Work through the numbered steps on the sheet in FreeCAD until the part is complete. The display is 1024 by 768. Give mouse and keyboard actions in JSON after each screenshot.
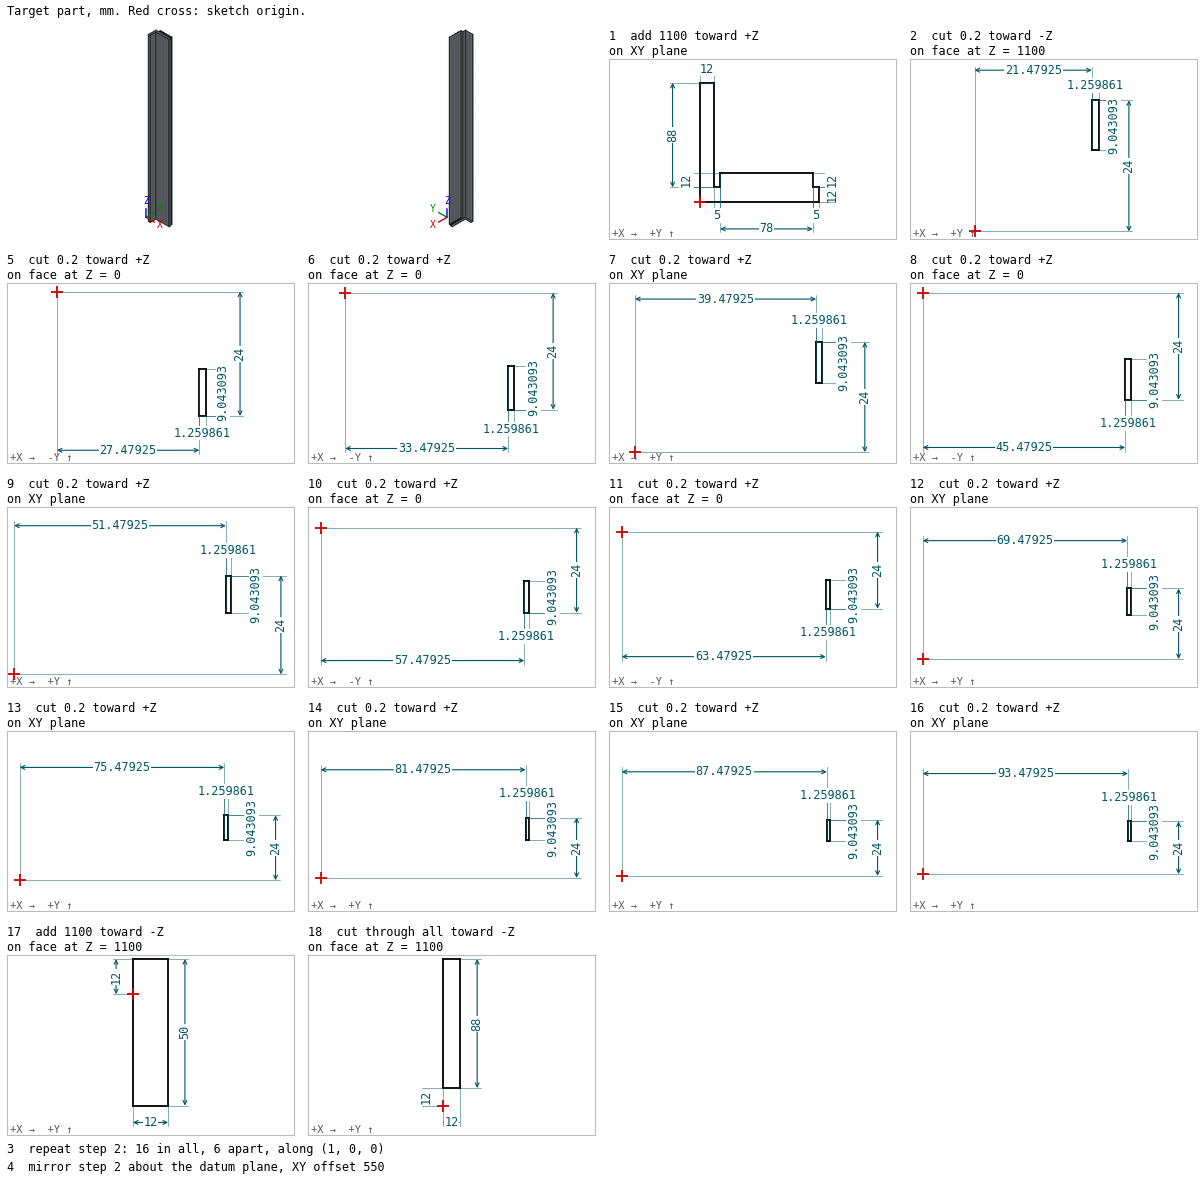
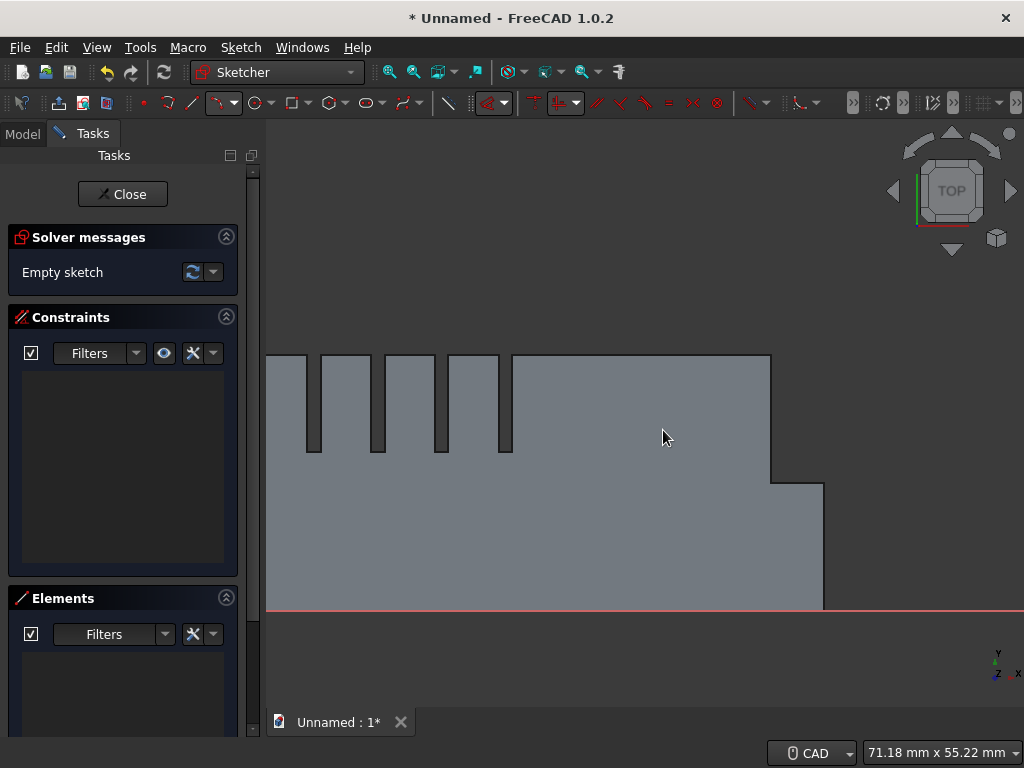
{"action": "scroll", "coordinate": [567, 400], "scroll_direction": "up", "scroll_amount": 7}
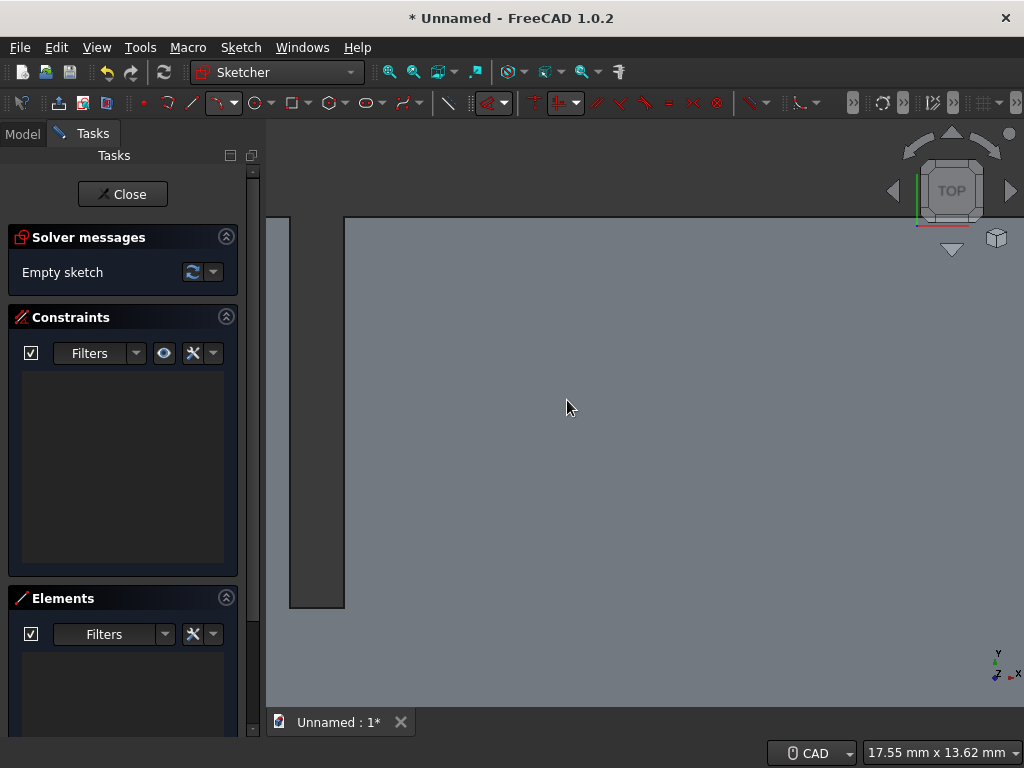
{"action": "left_click", "coordinate": [292, 104]}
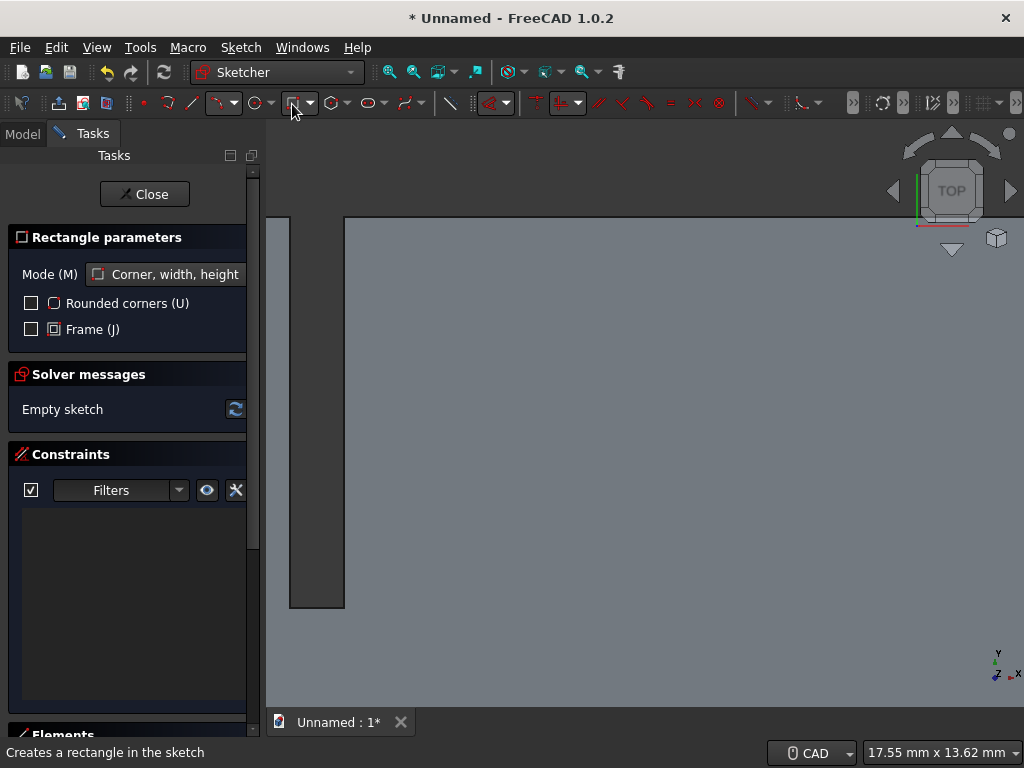
{"action": "left_click", "coordinate": [549, 217]}
{"action": "mouse_move", "coordinate": [603, 608]}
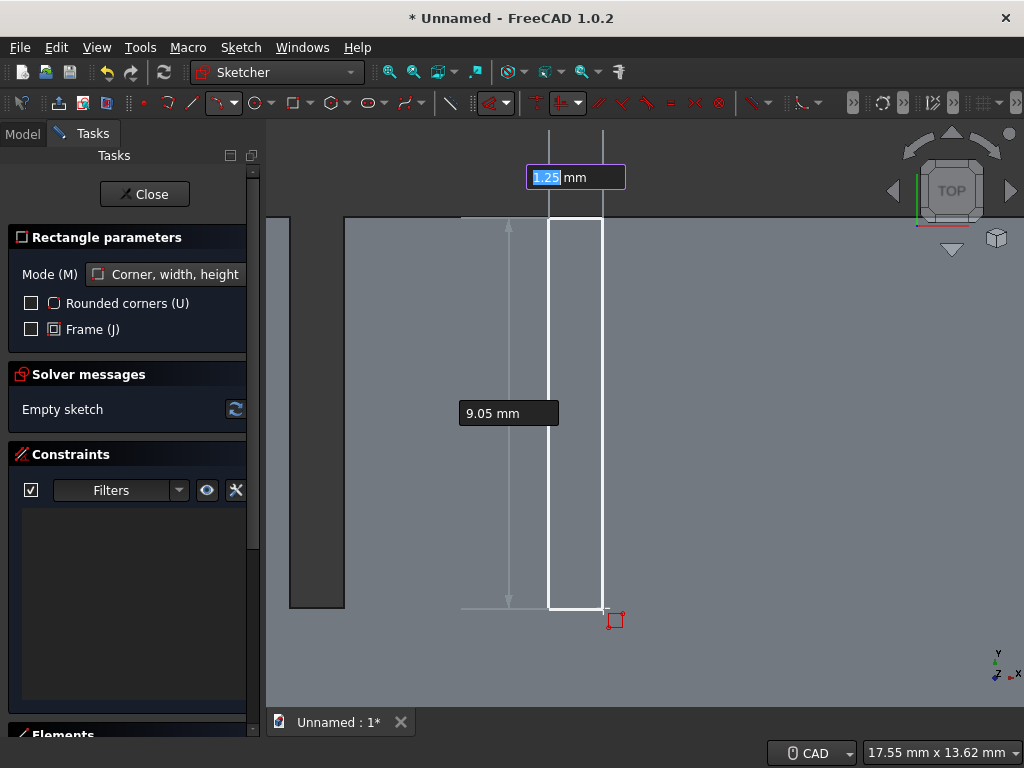
{"action": "type", "text": "1.259861"}
{"action": "key", "text": "Tab"}
{"action": "type", "text": "9.043093"}
{"action": "key", "text": "Return"}
{"action": "key", "text": "Escape"}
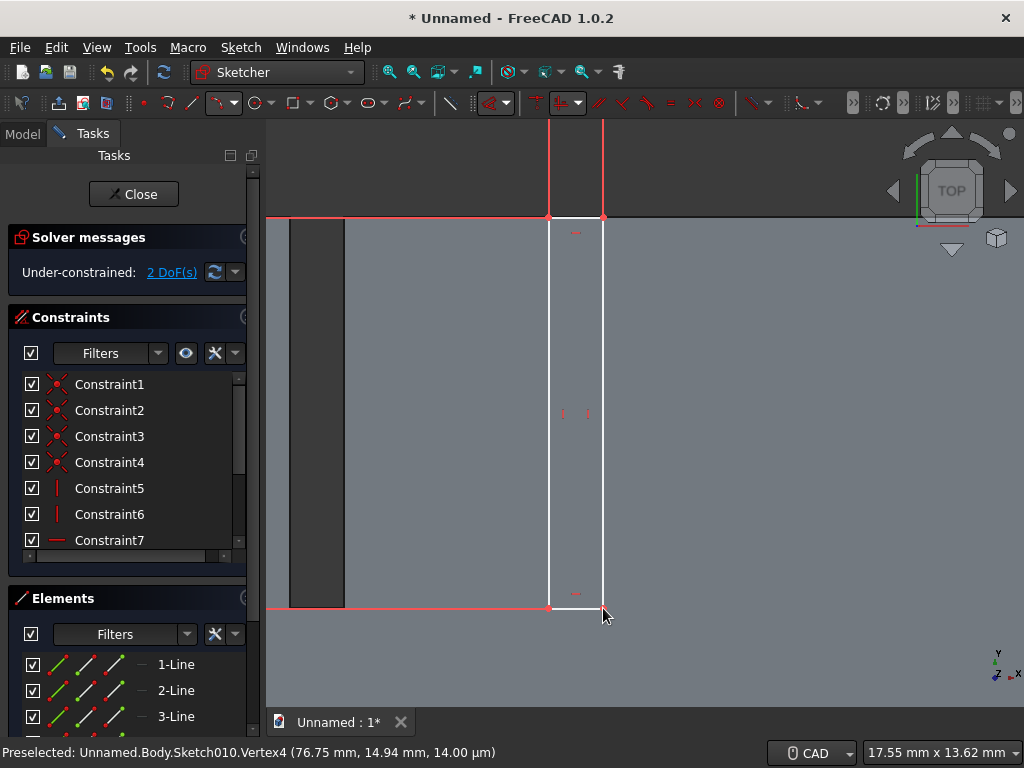
{"action": "left_click", "coordinate": [549, 218]}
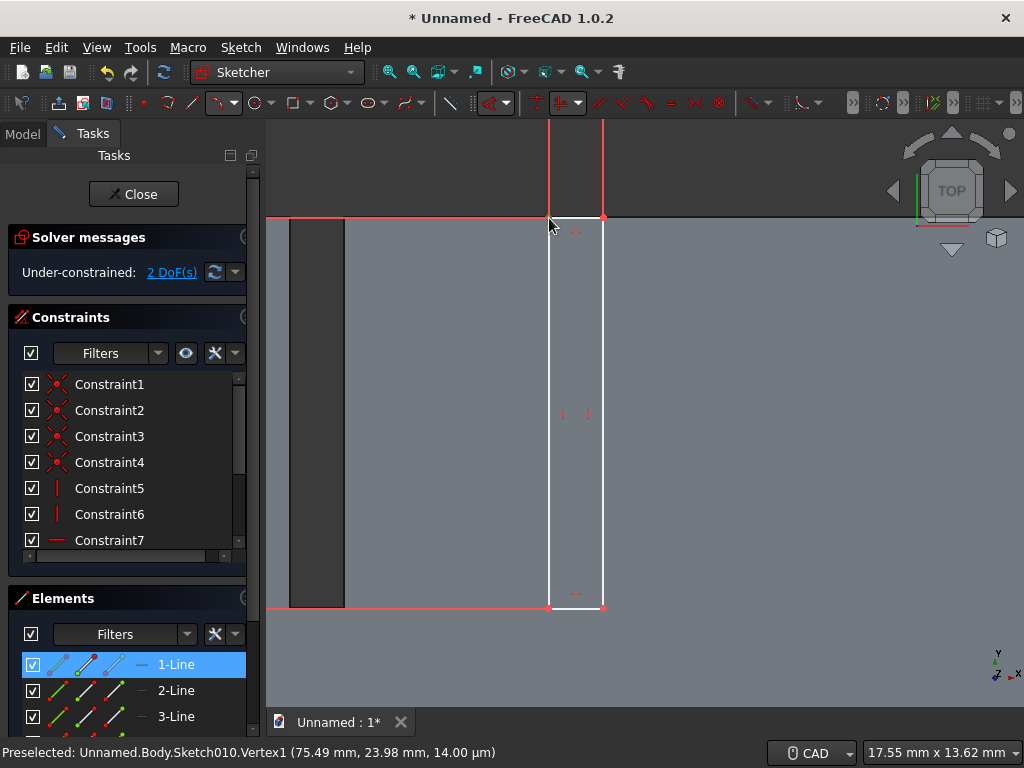
{"action": "key", "text": "i"}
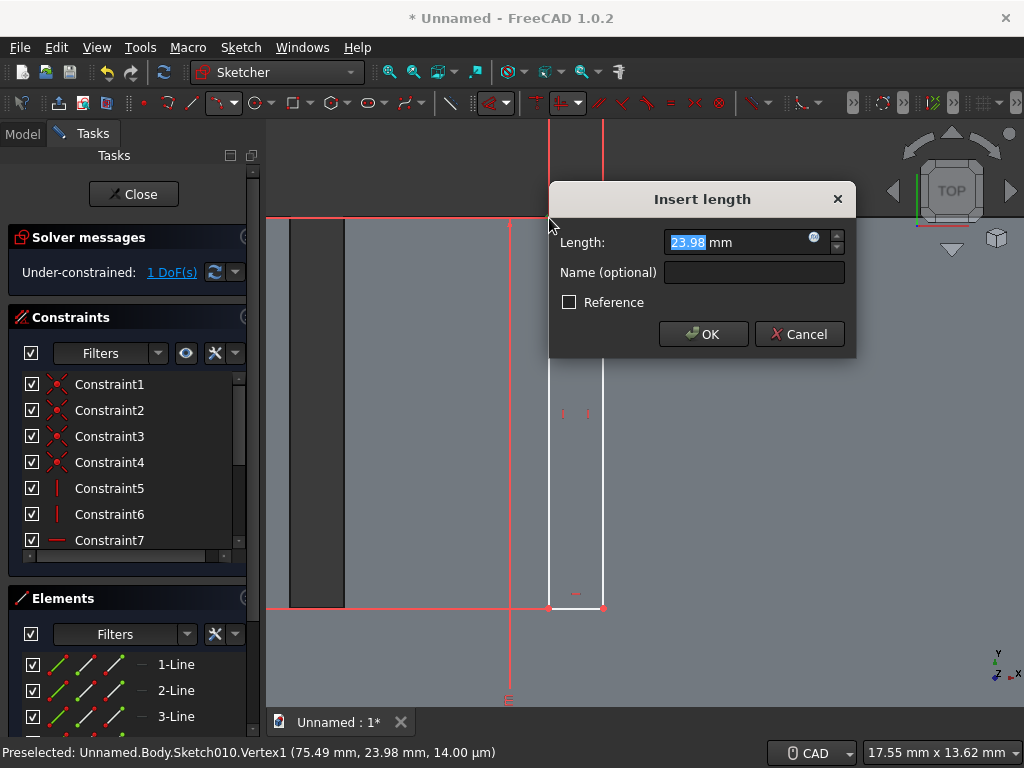
{"action": "type", "text": "24"}
{"action": "key", "text": "Return"}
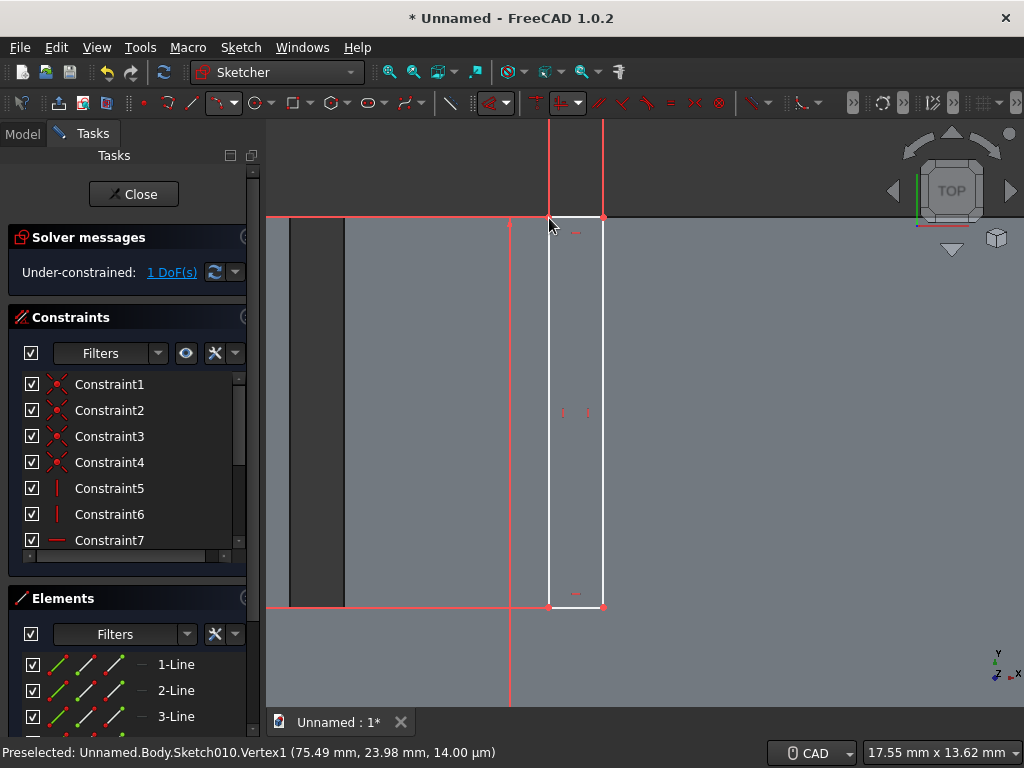
{"action": "left_click", "coordinate": [549, 217]}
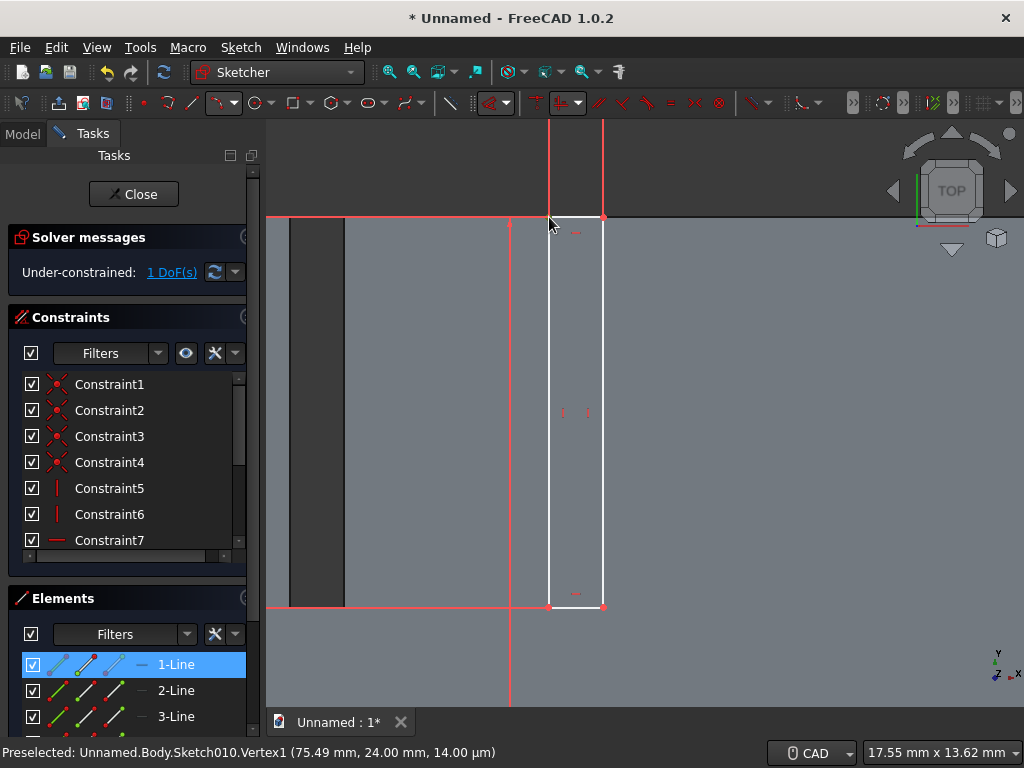
{"action": "left_click", "coordinate": [508, 104]}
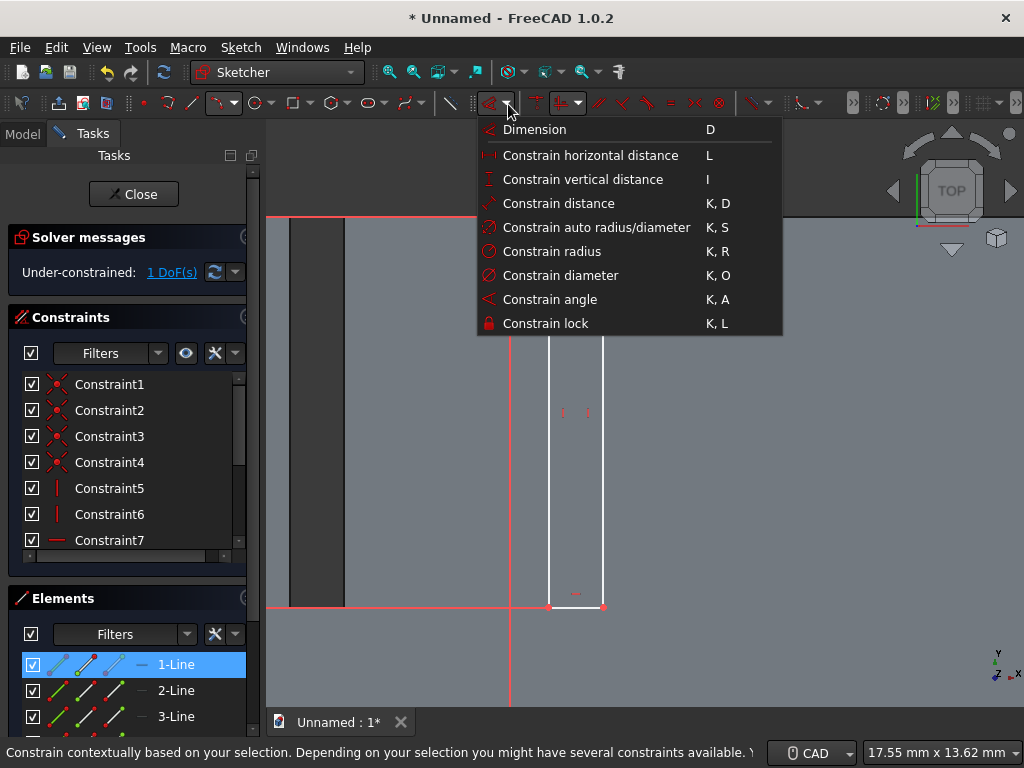
{"action": "left_click", "coordinate": [630, 155]}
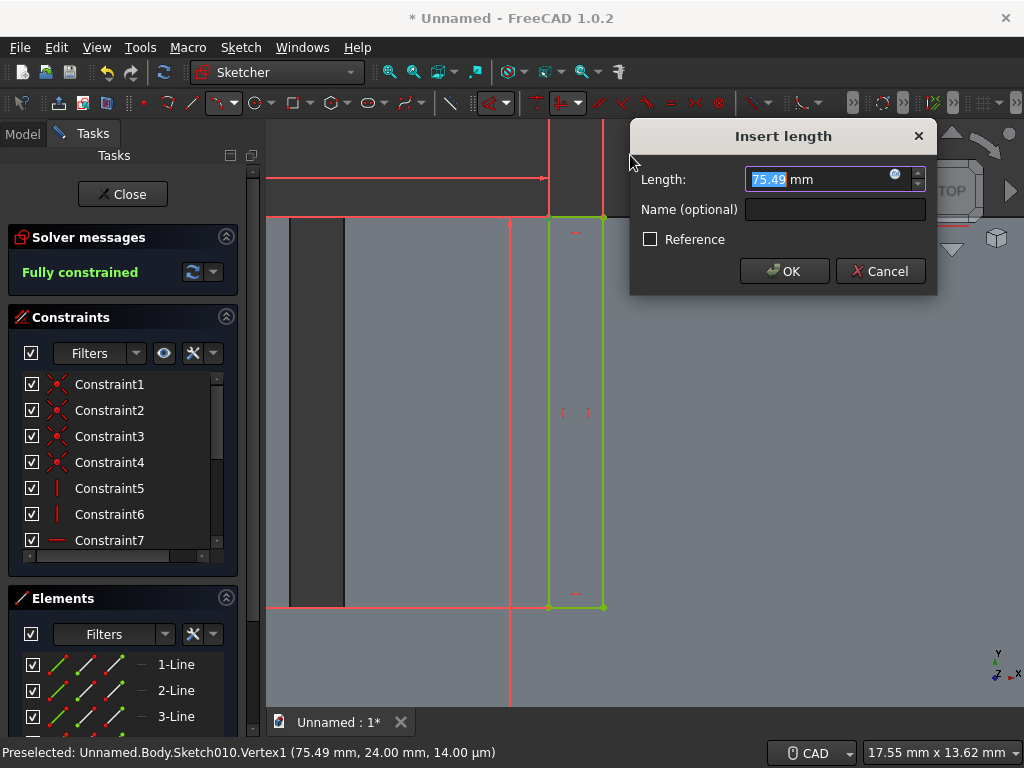
{"action": "type", "text": "75.47925"}
{"action": "key", "text": "Return"}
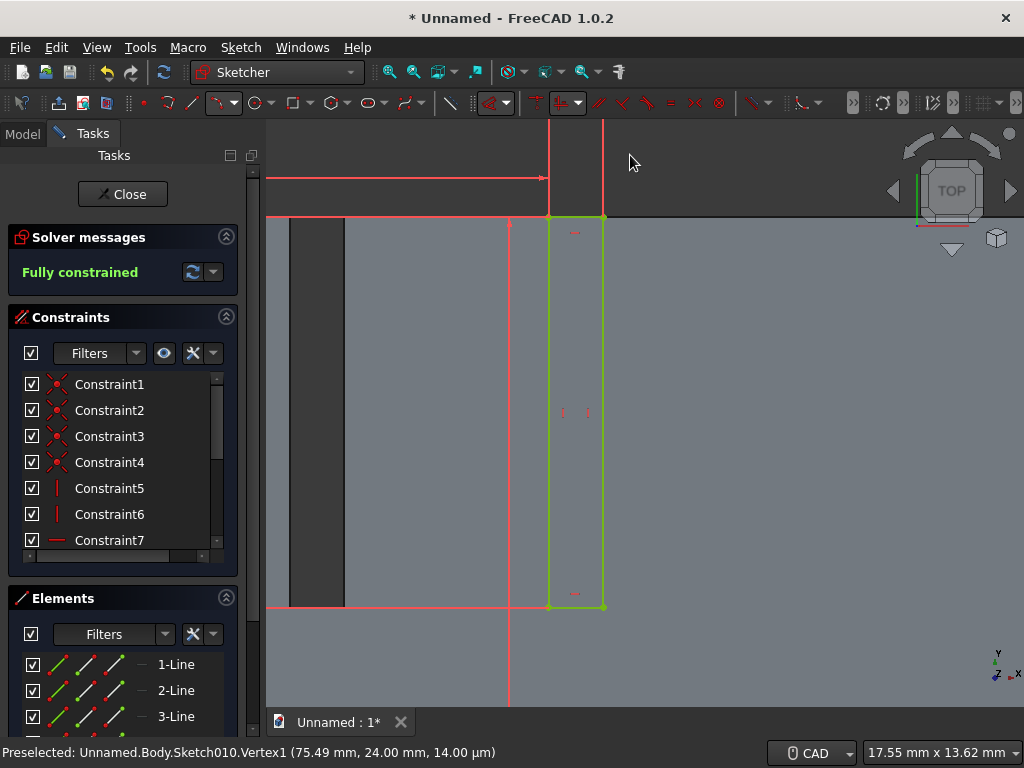
{"action": "left_click", "coordinate": [123, 194]}